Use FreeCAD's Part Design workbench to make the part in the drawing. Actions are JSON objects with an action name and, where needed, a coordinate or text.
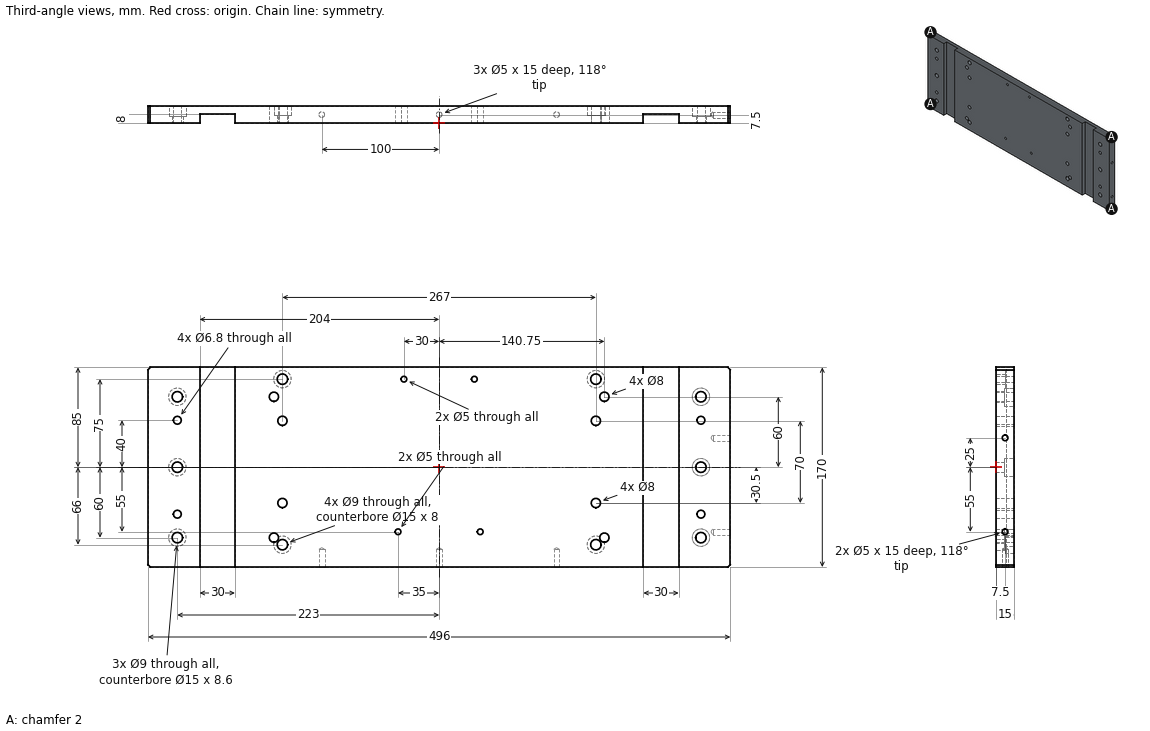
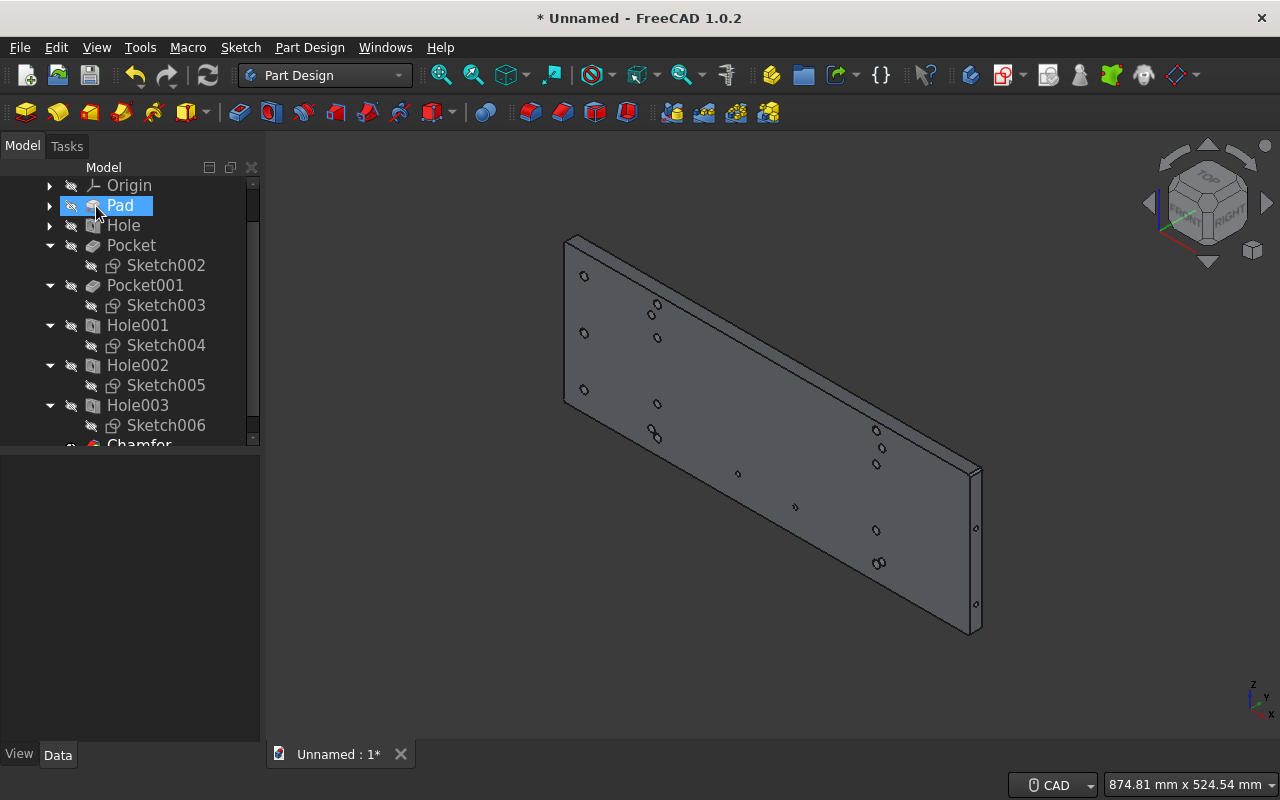
{"action": "left_click", "coordinate": [825, 471]}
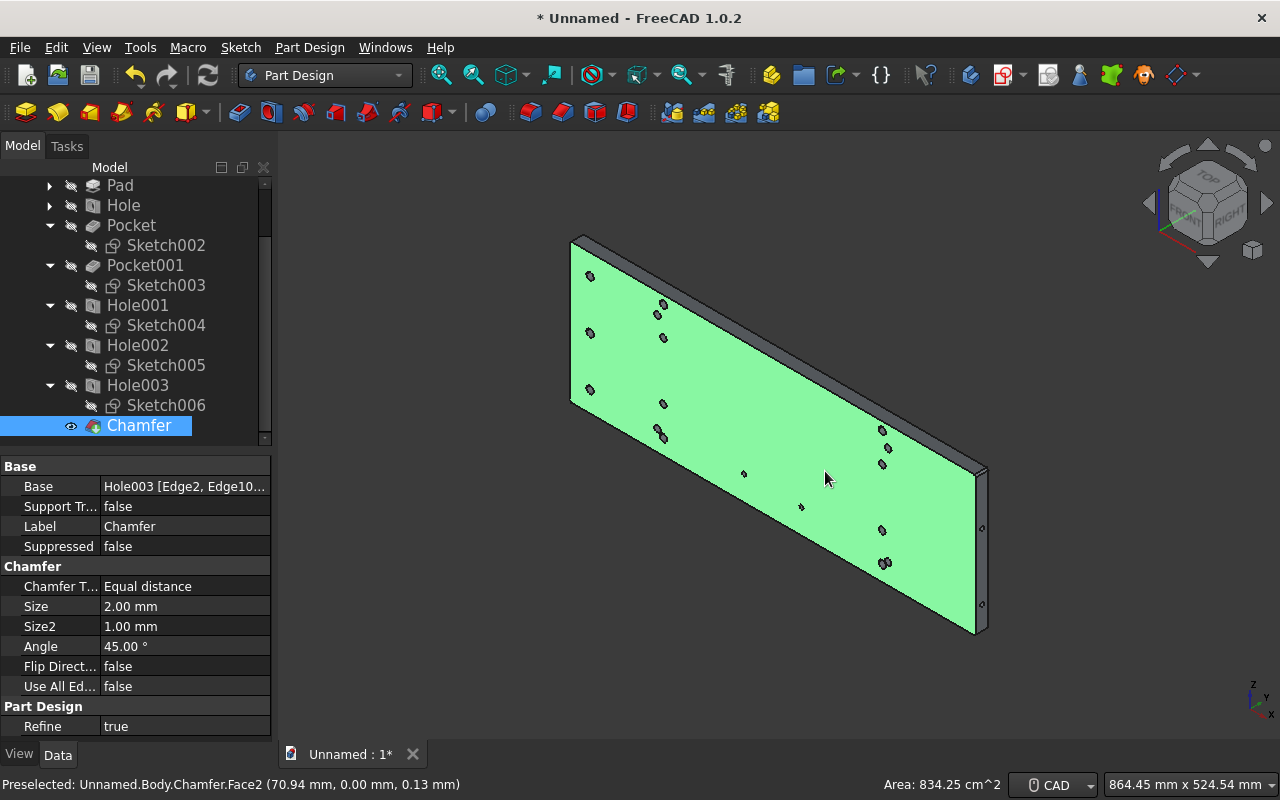
{"action": "left_click", "coordinate": [1004, 76]}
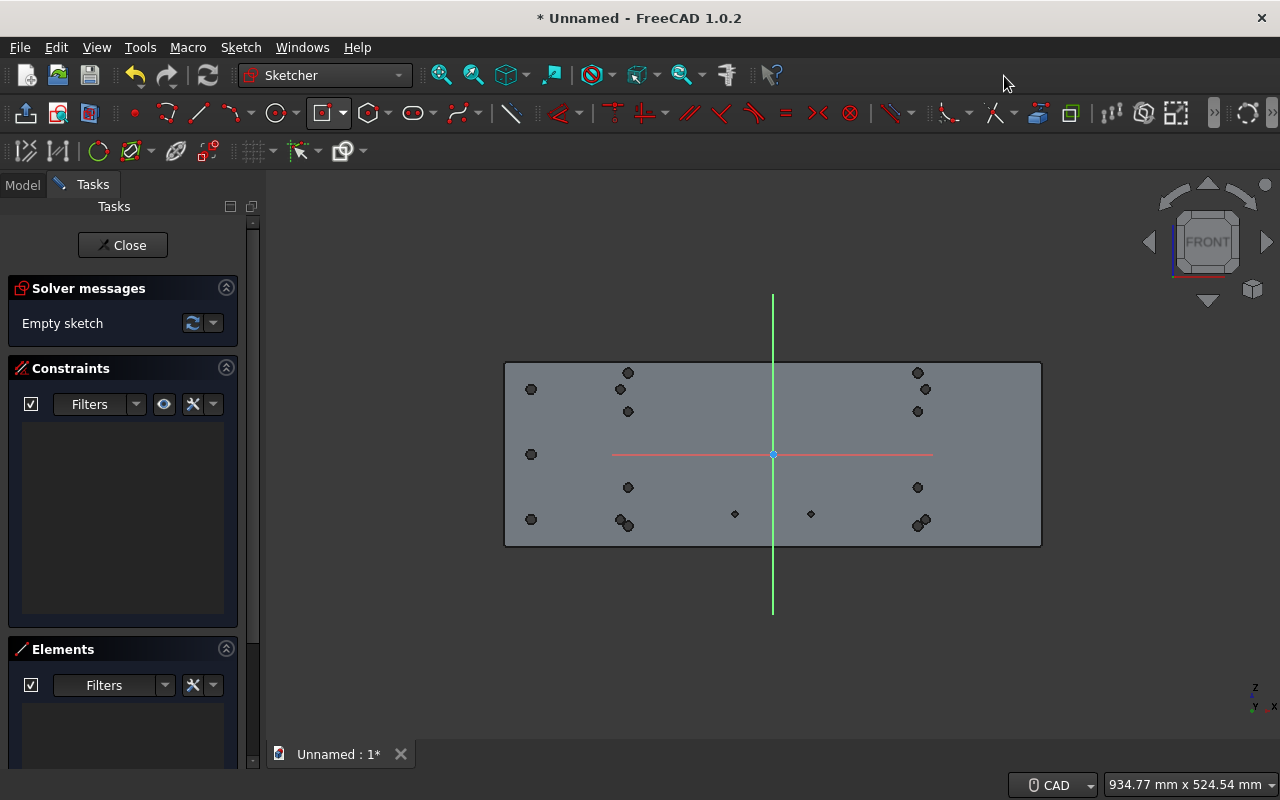
{"action": "scroll", "coordinate": [795, 399], "scroll_direction": "up", "scroll_amount": 7}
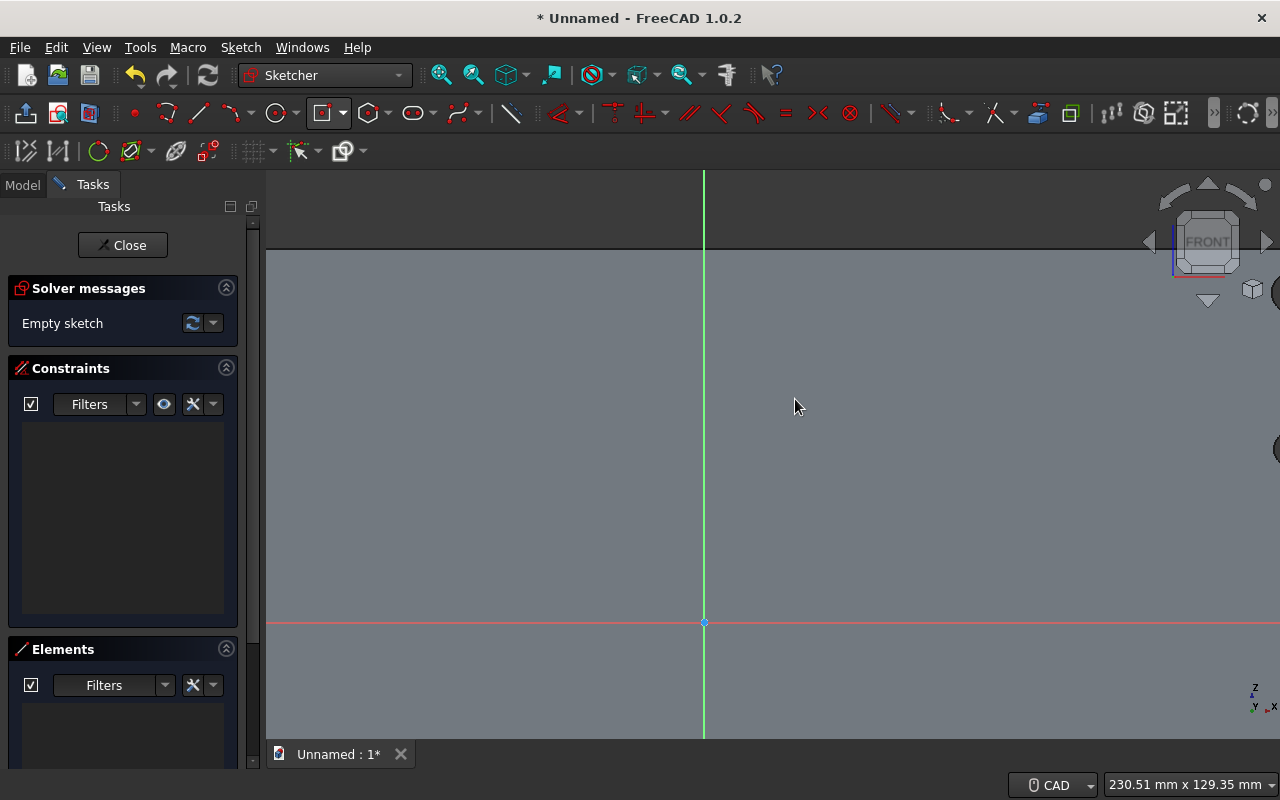
{"action": "left_click", "coordinate": [276, 114]}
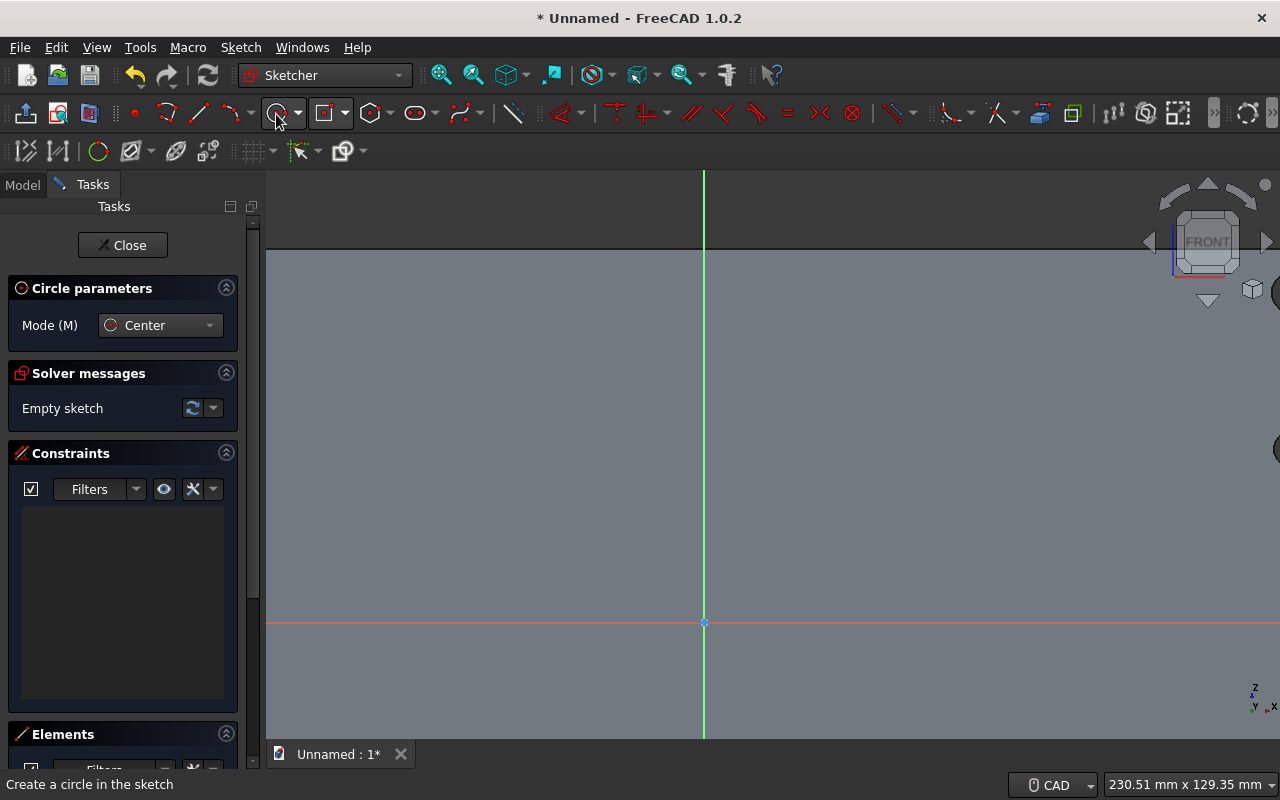
{"action": "scroll", "coordinate": [572, 293], "scroll_direction": "up", "scroll_amount": 4}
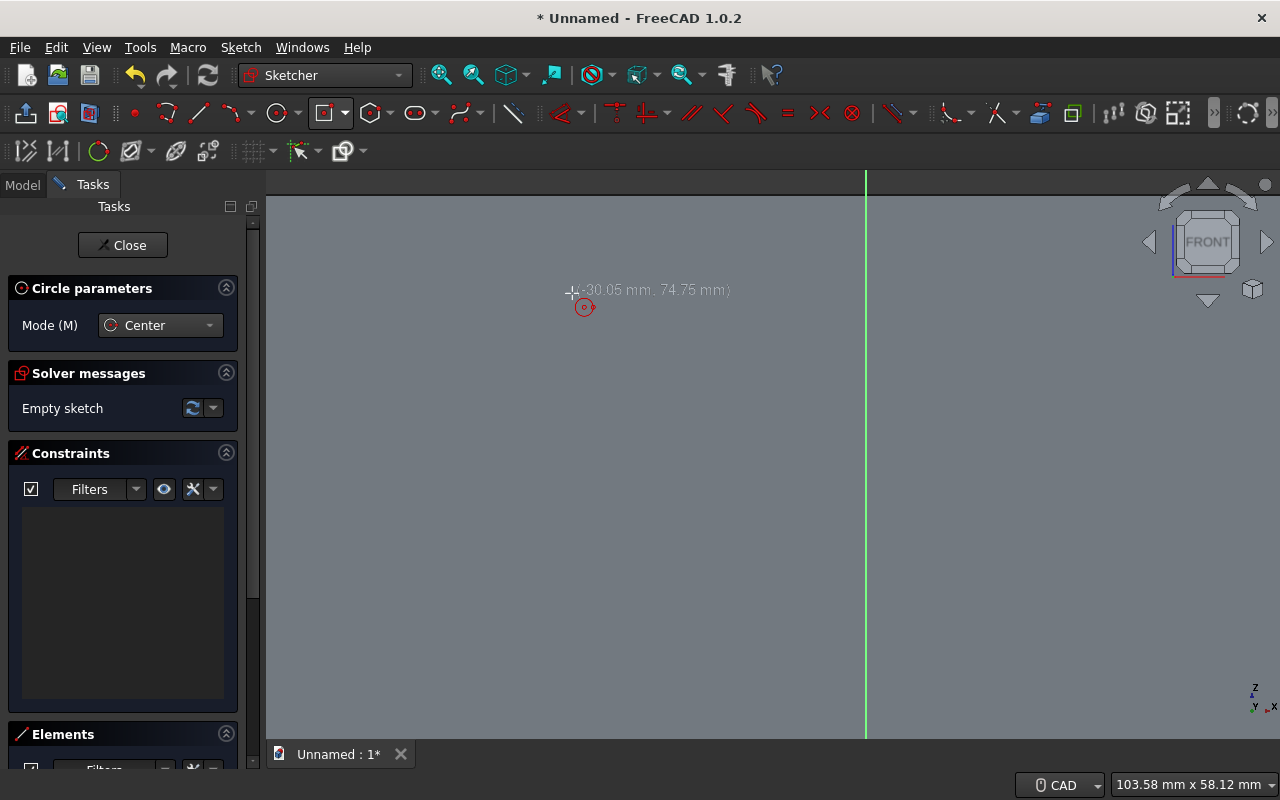
{"action": "left_click", "coordinate": [572, 293]}
{"action": "mouse_move", "coordinate": [589, 275]}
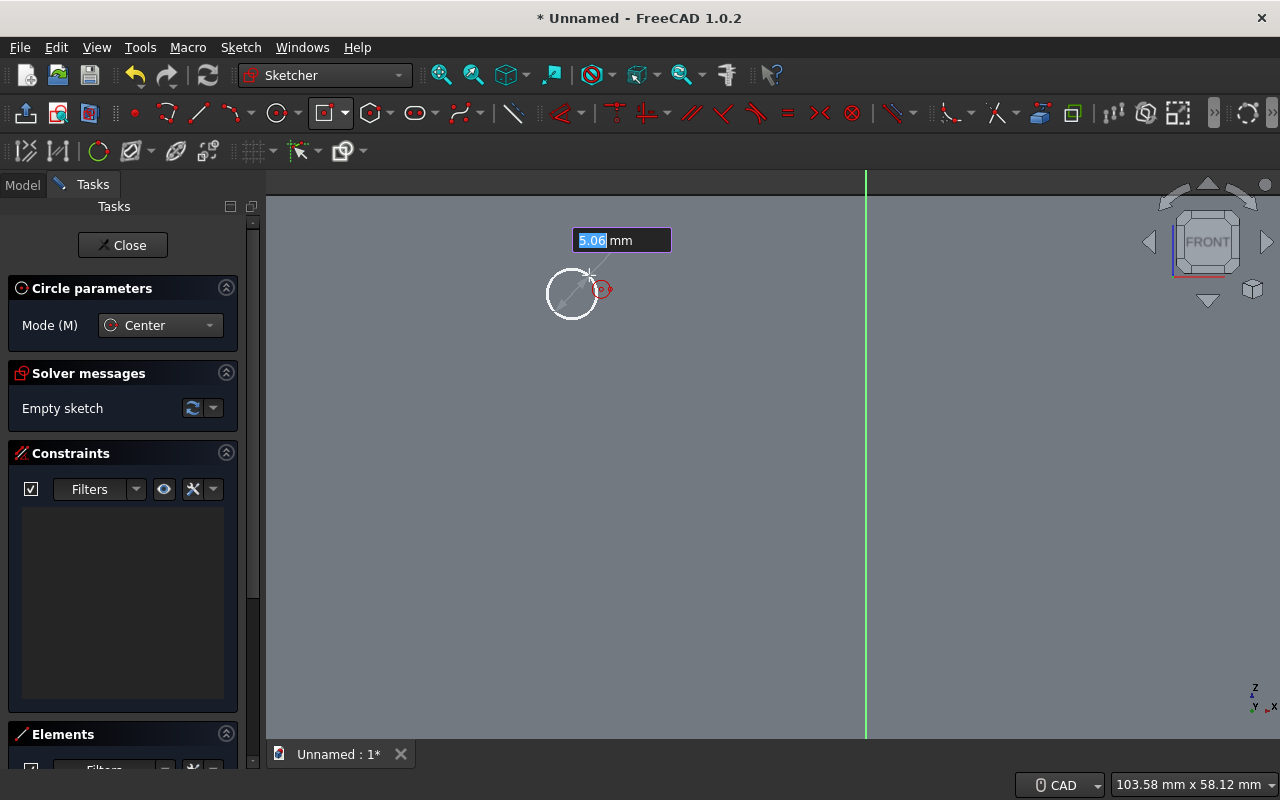
{"action": "type", "text": "5"}
{"action": "key", "text": "Return"}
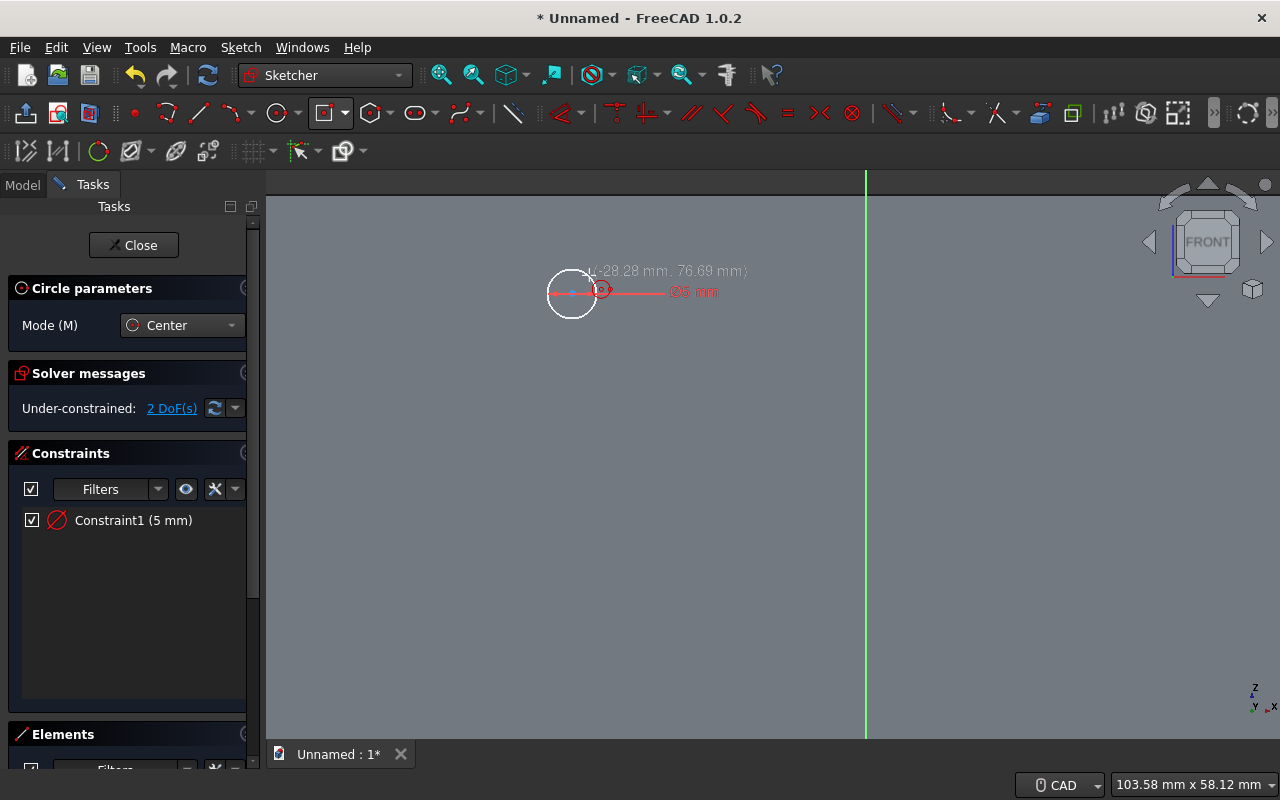
{"action": "scroll", "coordinate": [573, 297], "scroll_direction": "down", "scroll_amount": 4}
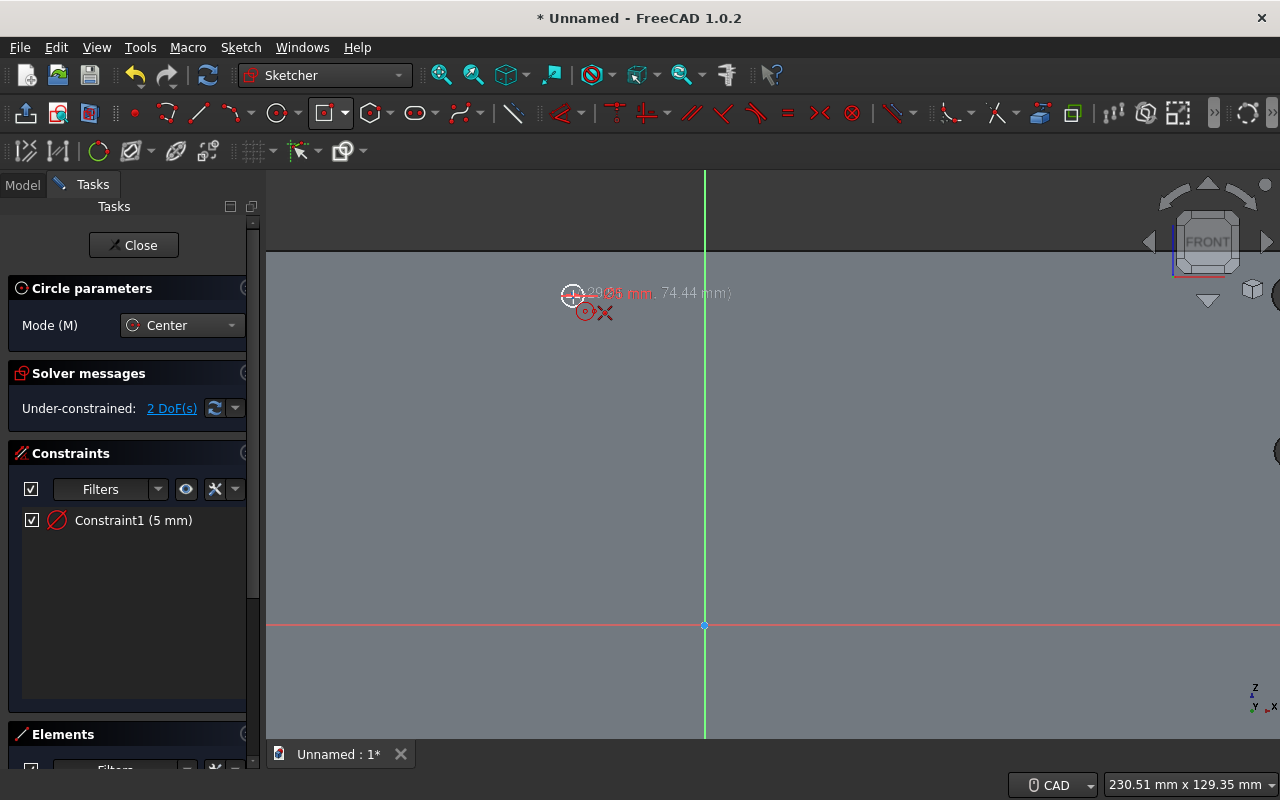
{"action": "scroll", "coordinate": [837, 295], "scroll_direction": "up", "scroll_amount": 4}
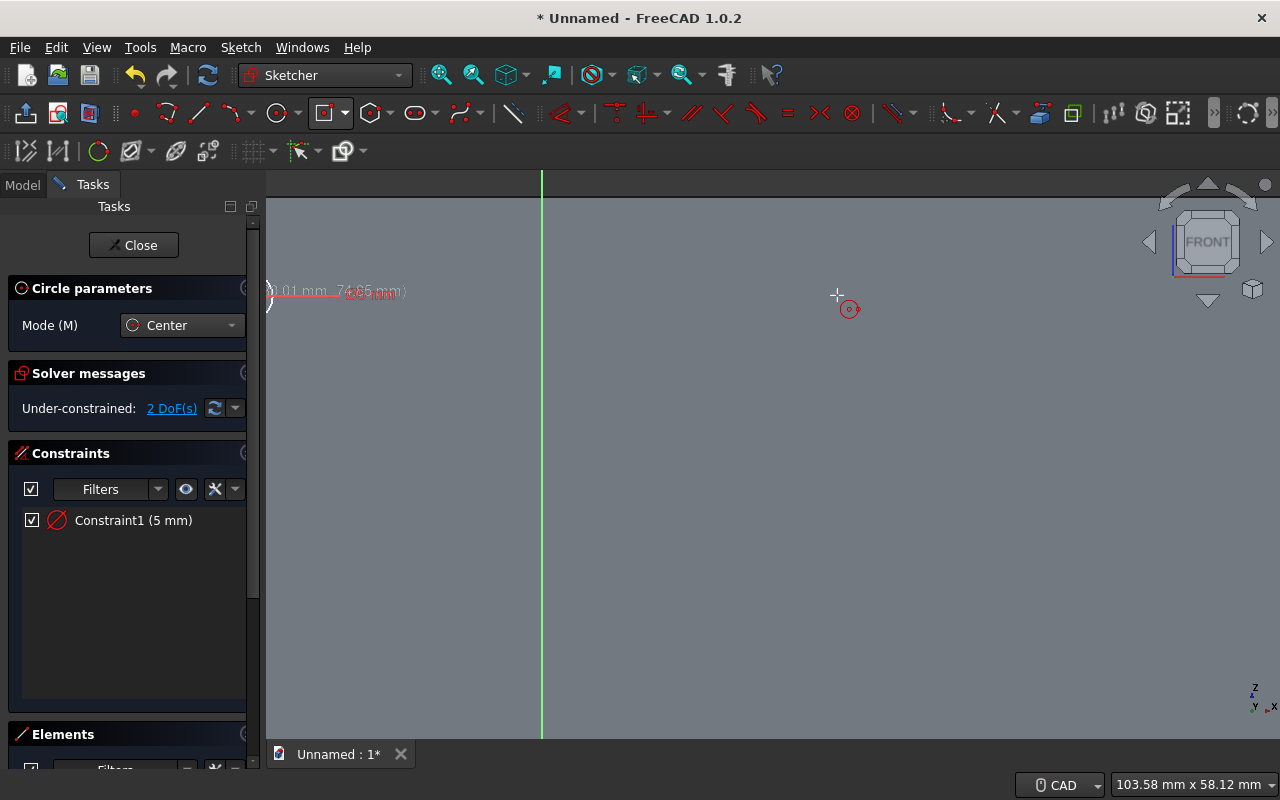
{"action": "left_click", "coordinate": [836, 295]}
{"action": "mouse_move", "coordinate": [853, 278]}